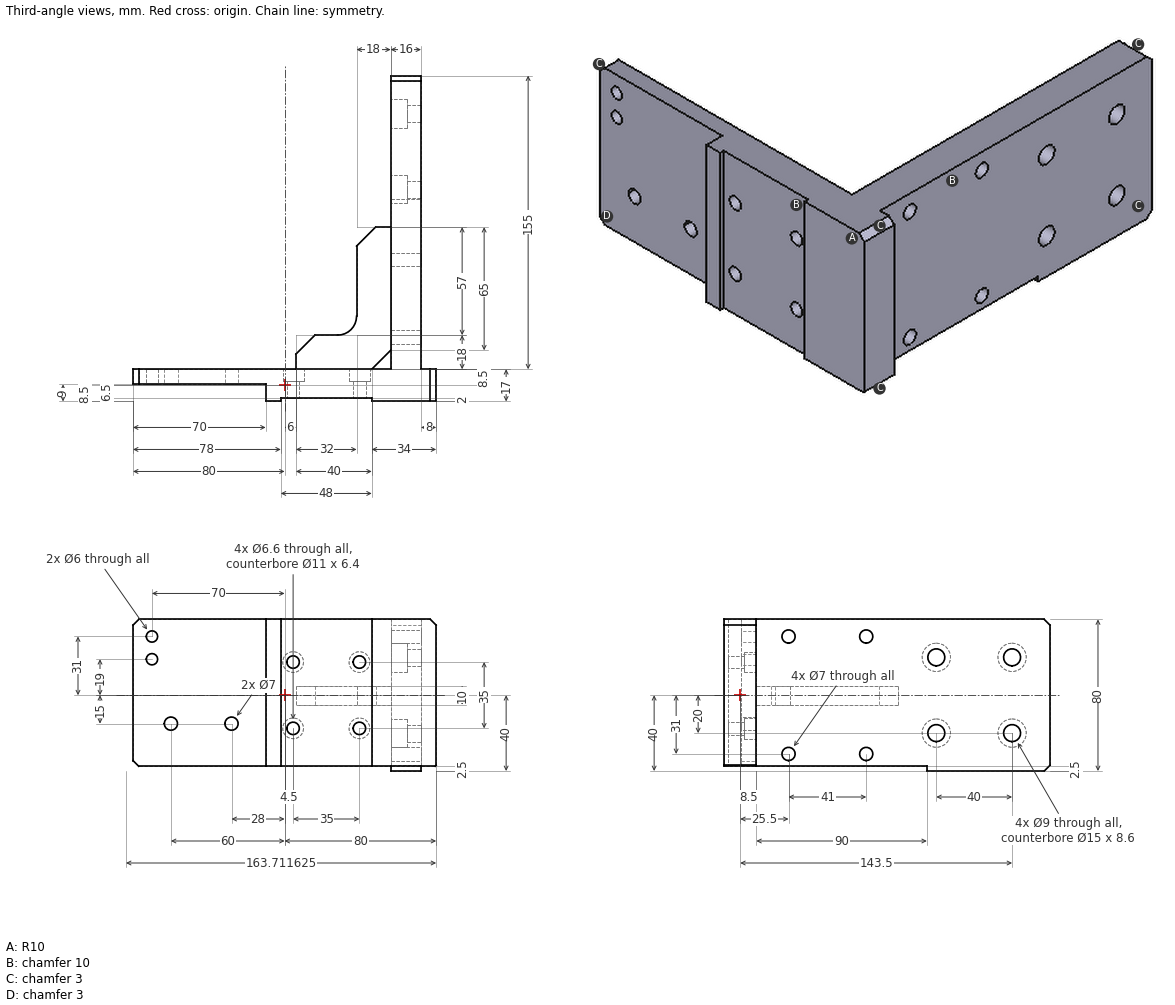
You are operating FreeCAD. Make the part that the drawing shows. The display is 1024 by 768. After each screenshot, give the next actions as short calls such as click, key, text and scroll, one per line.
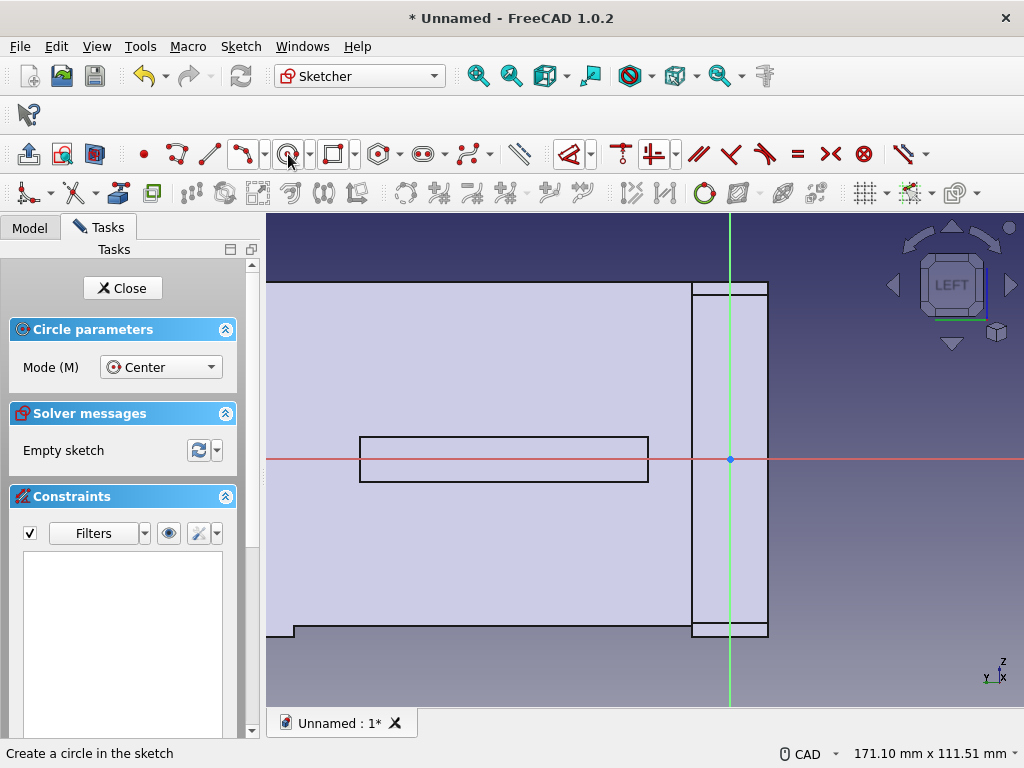
scroll(617, 597, up, 2)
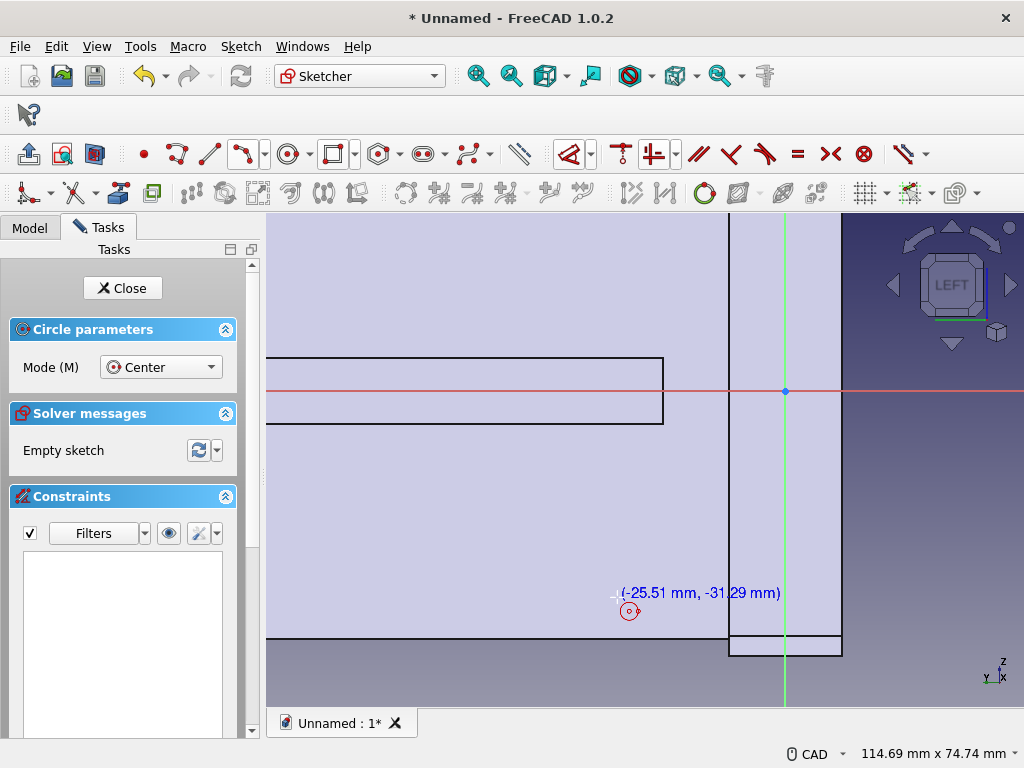
click(617, 596)
click(633, 580)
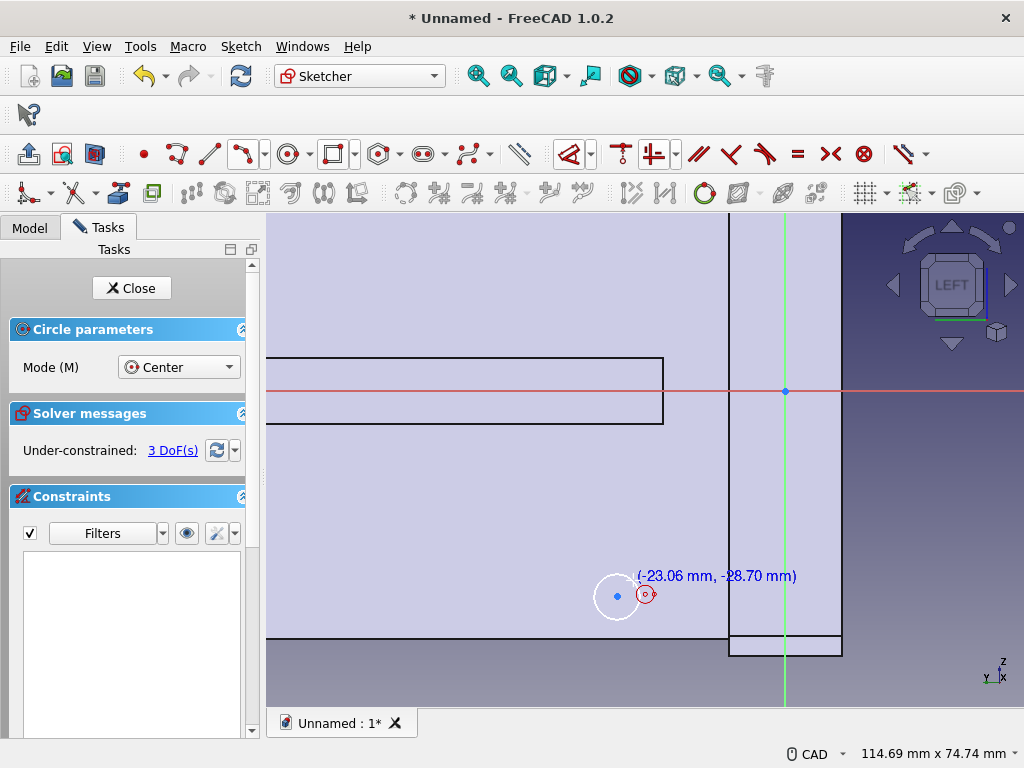
click(346, 596)
click(362, 580)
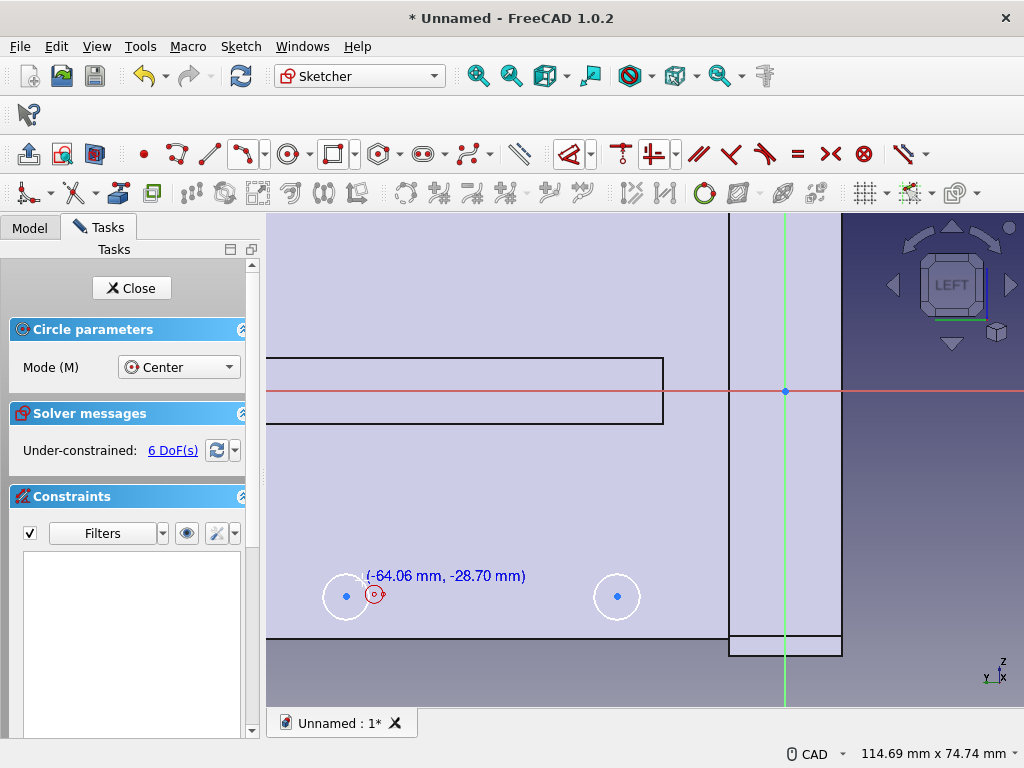
scroll(622, 600, down, 2)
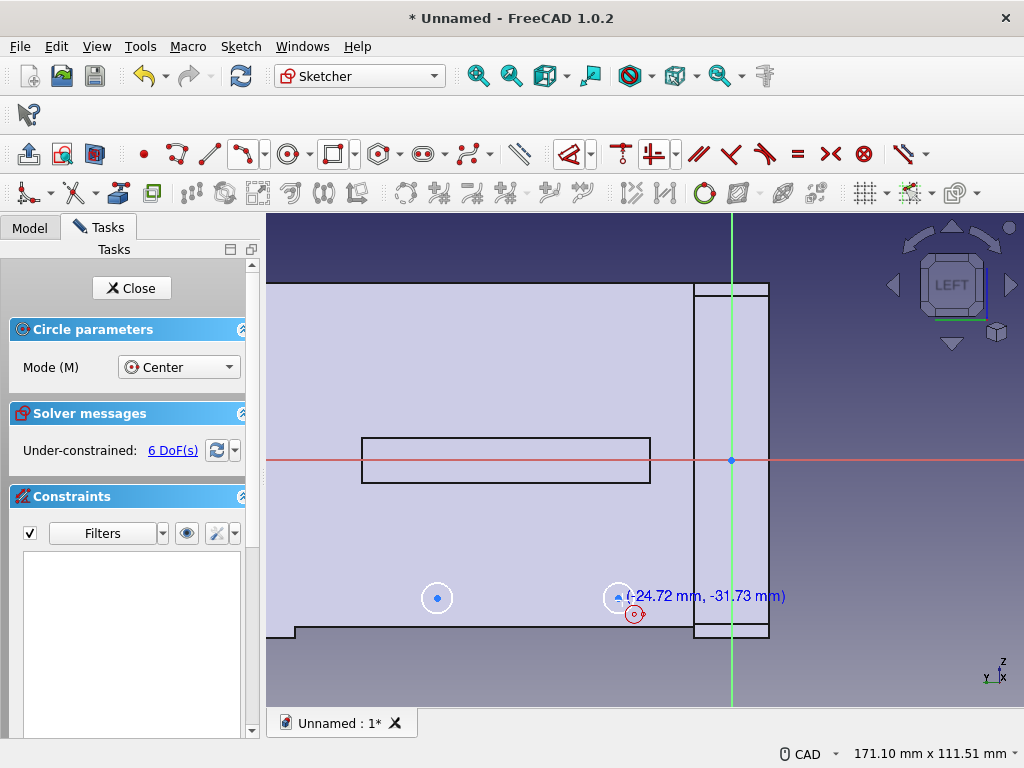
scroll(437, 323, up, 2)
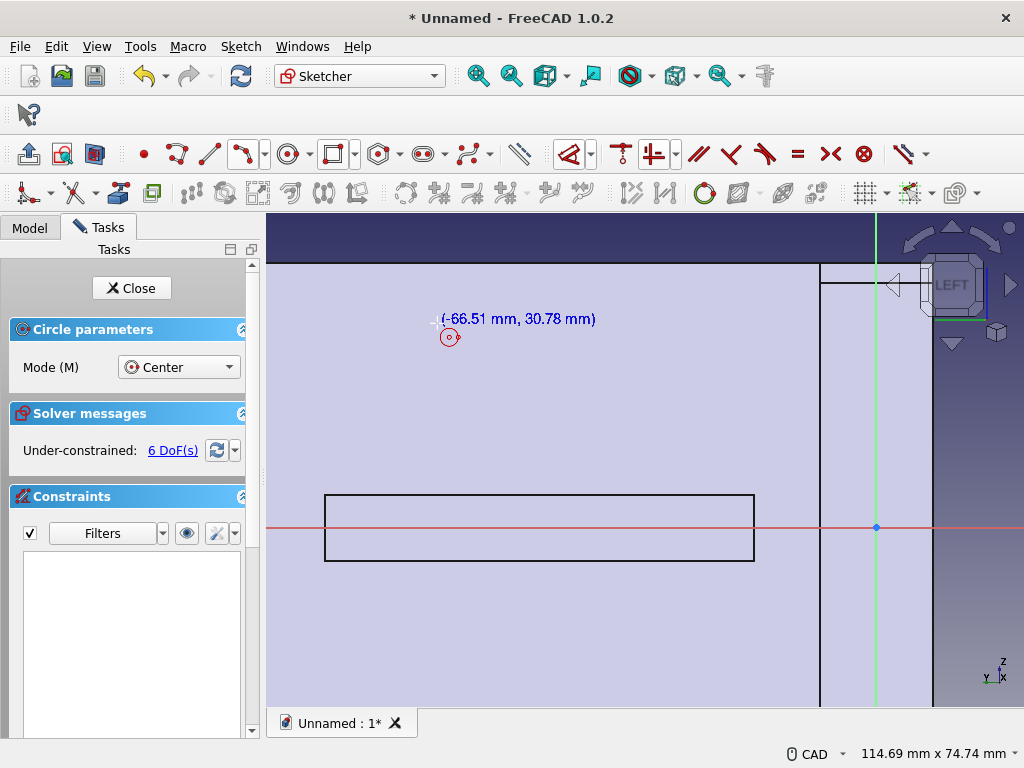
click(437, 323)
click(453, 307)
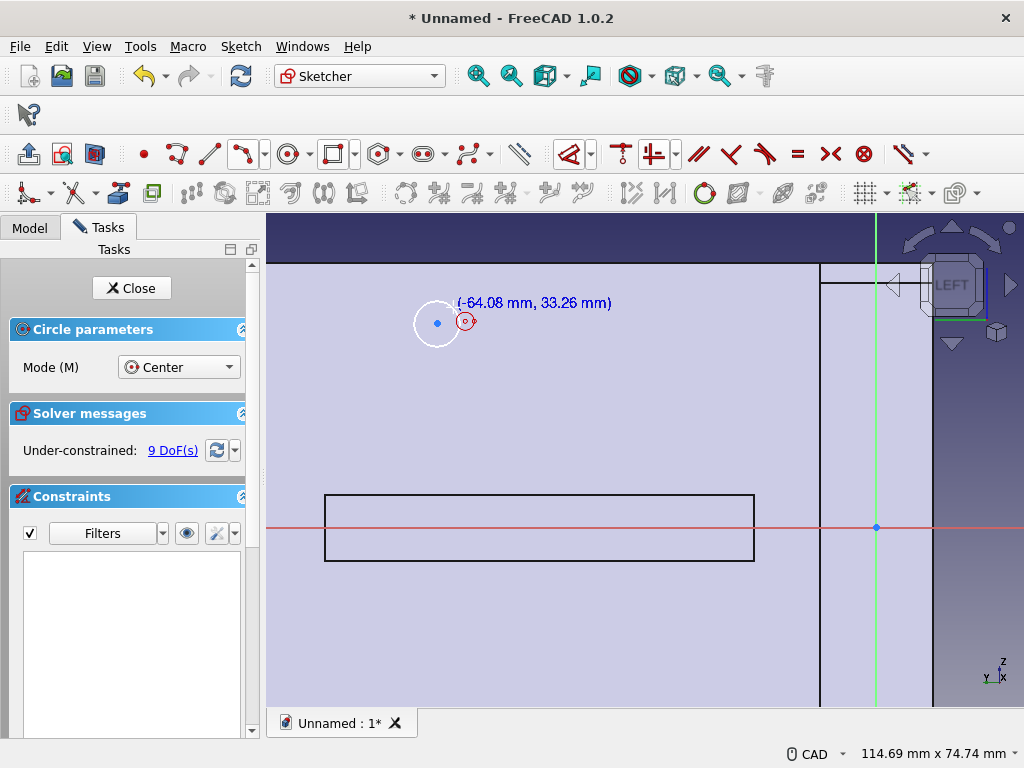
click(708, 323)
click(724, 307)
key(Escape)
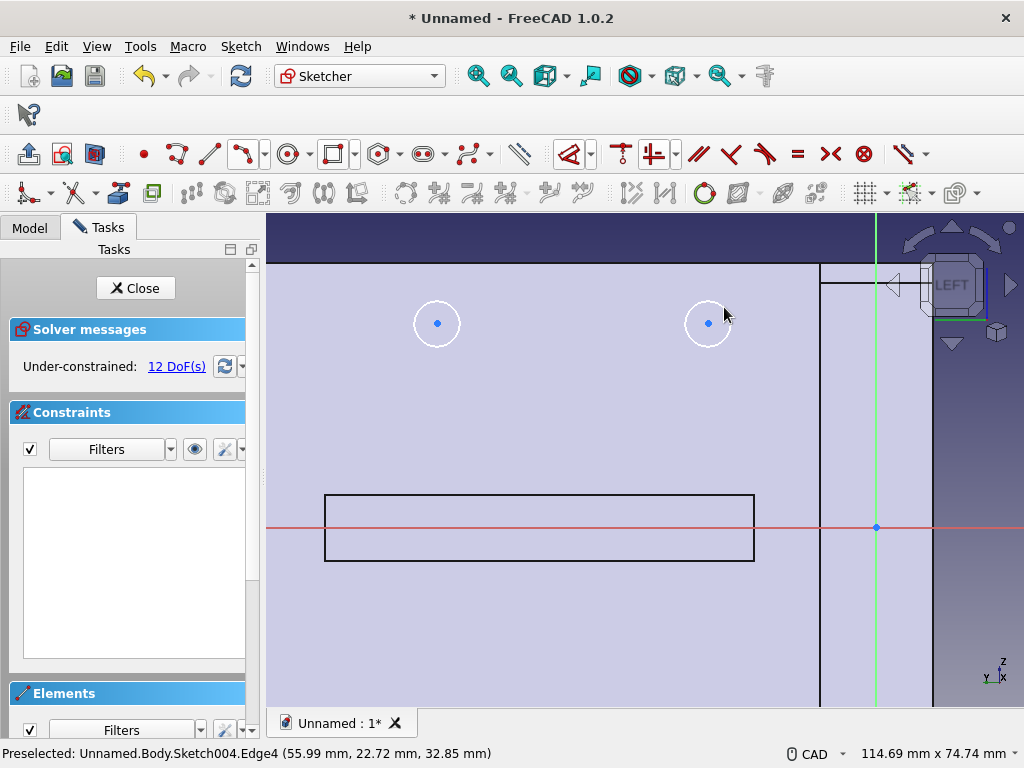
scroll(437, 322, down, 2)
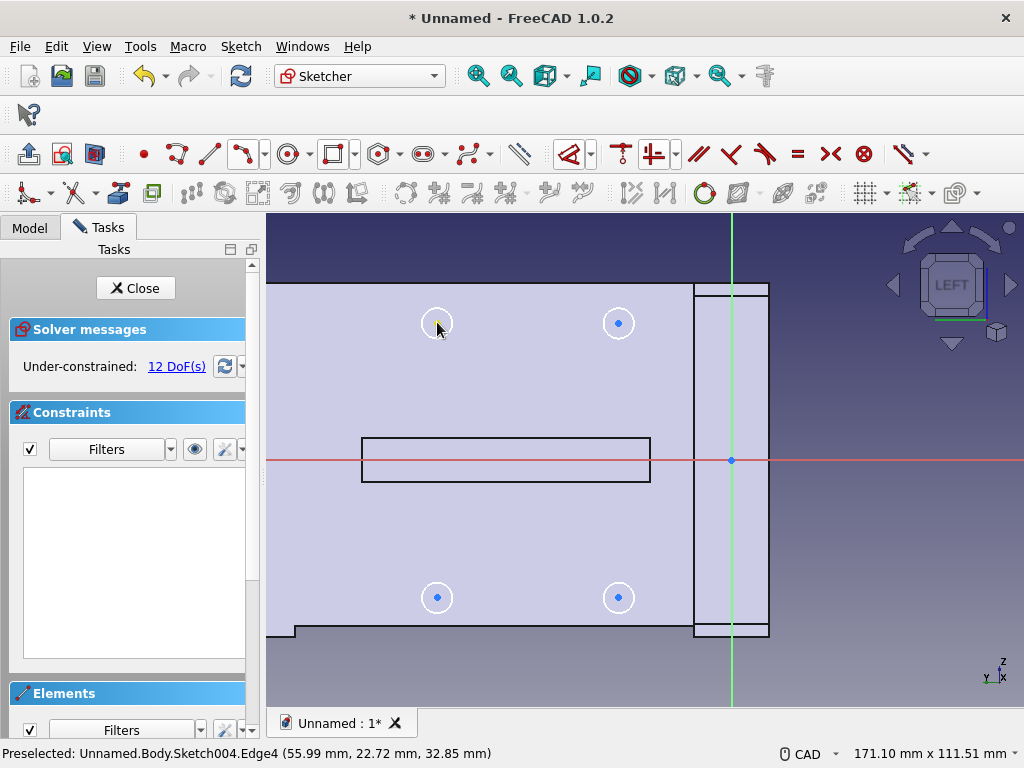
click(629, 587)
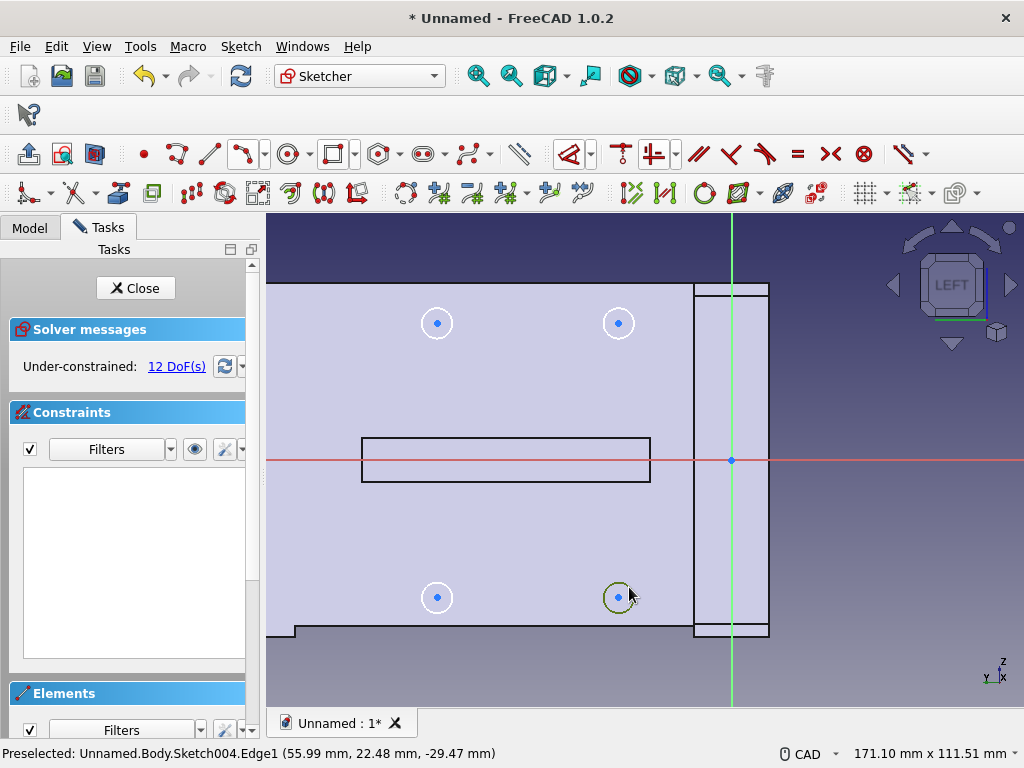
click(448, 587)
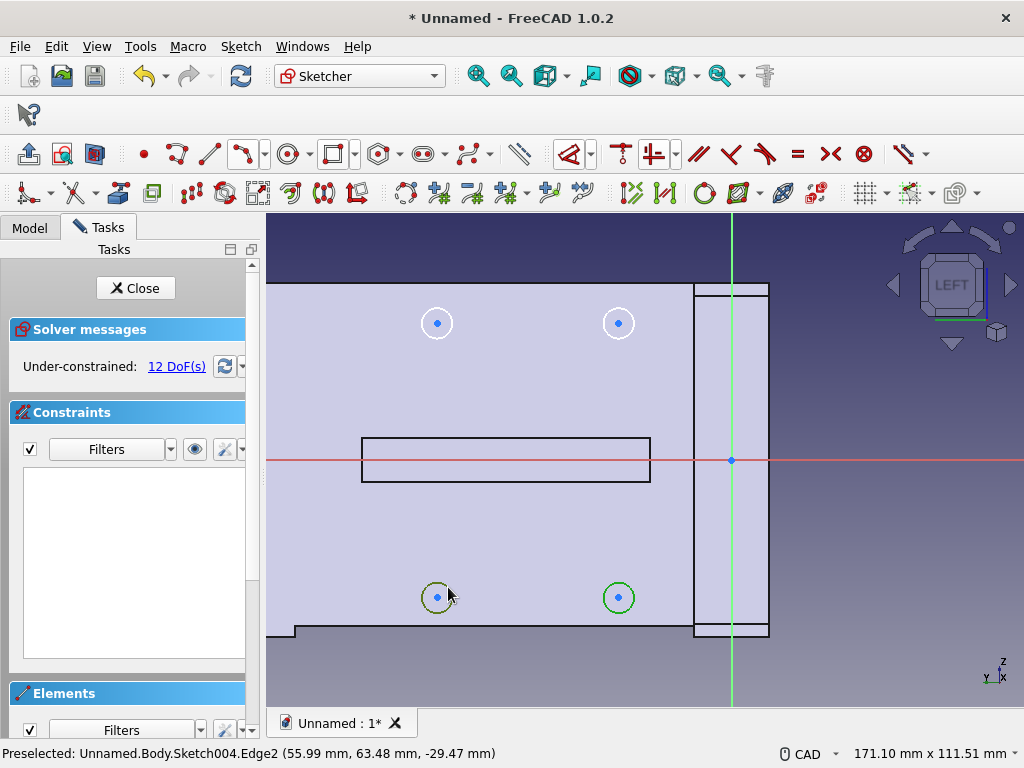
click(448, 313)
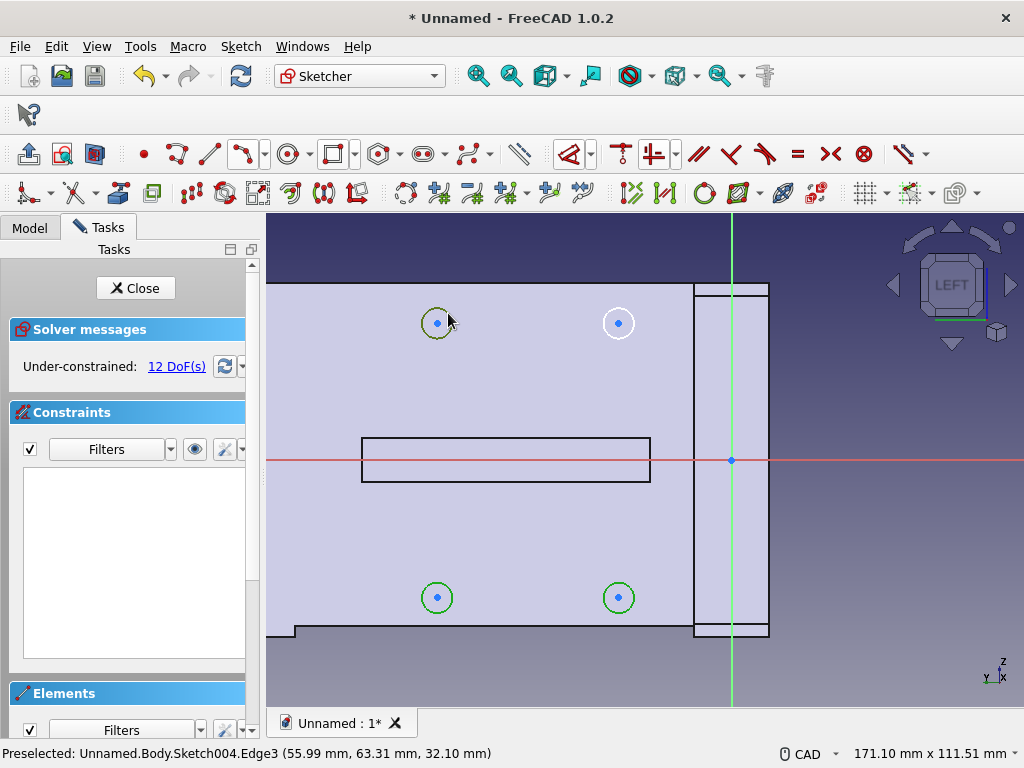
click(629, 313)